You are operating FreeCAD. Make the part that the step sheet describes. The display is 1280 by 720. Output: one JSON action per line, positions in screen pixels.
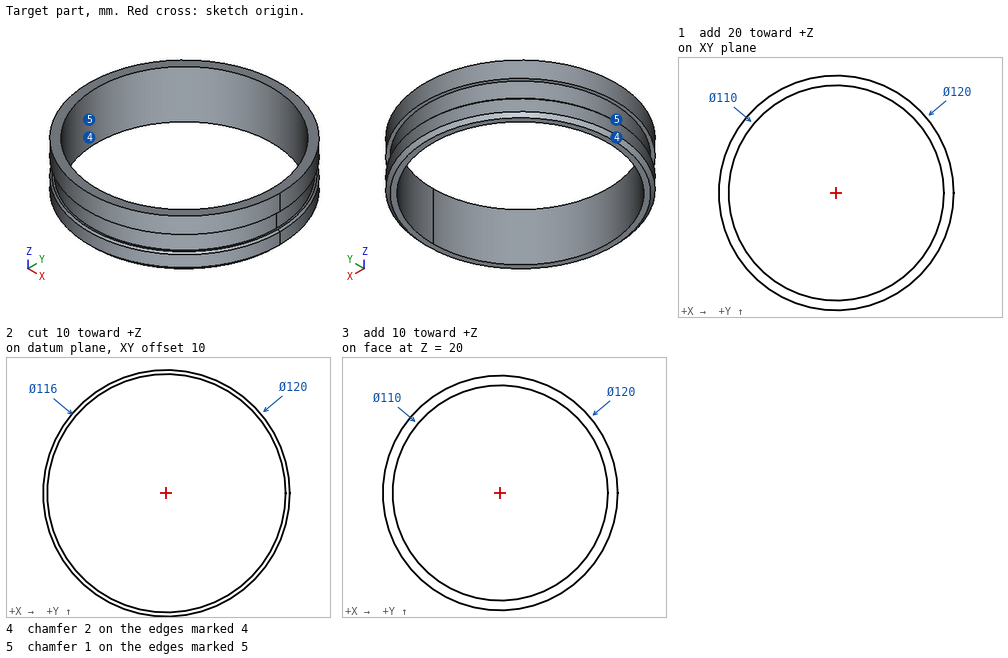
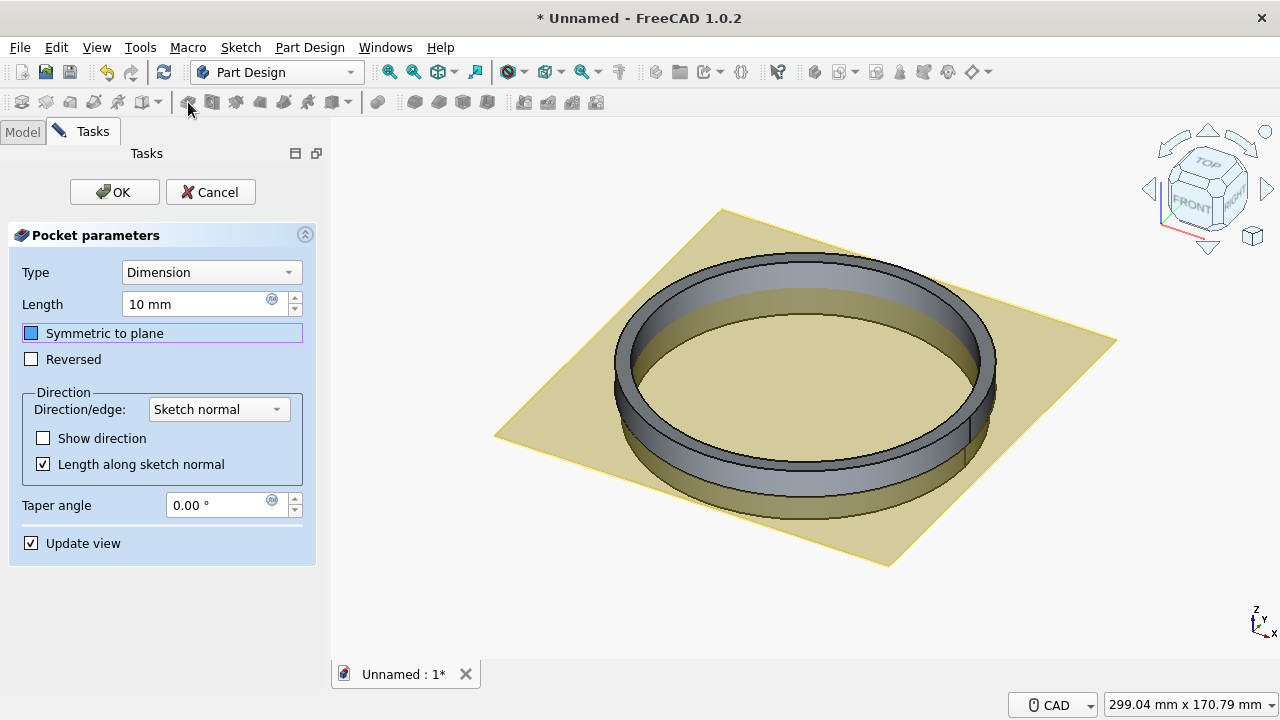
{"action": "left_click", "coordinate": [30, 359]}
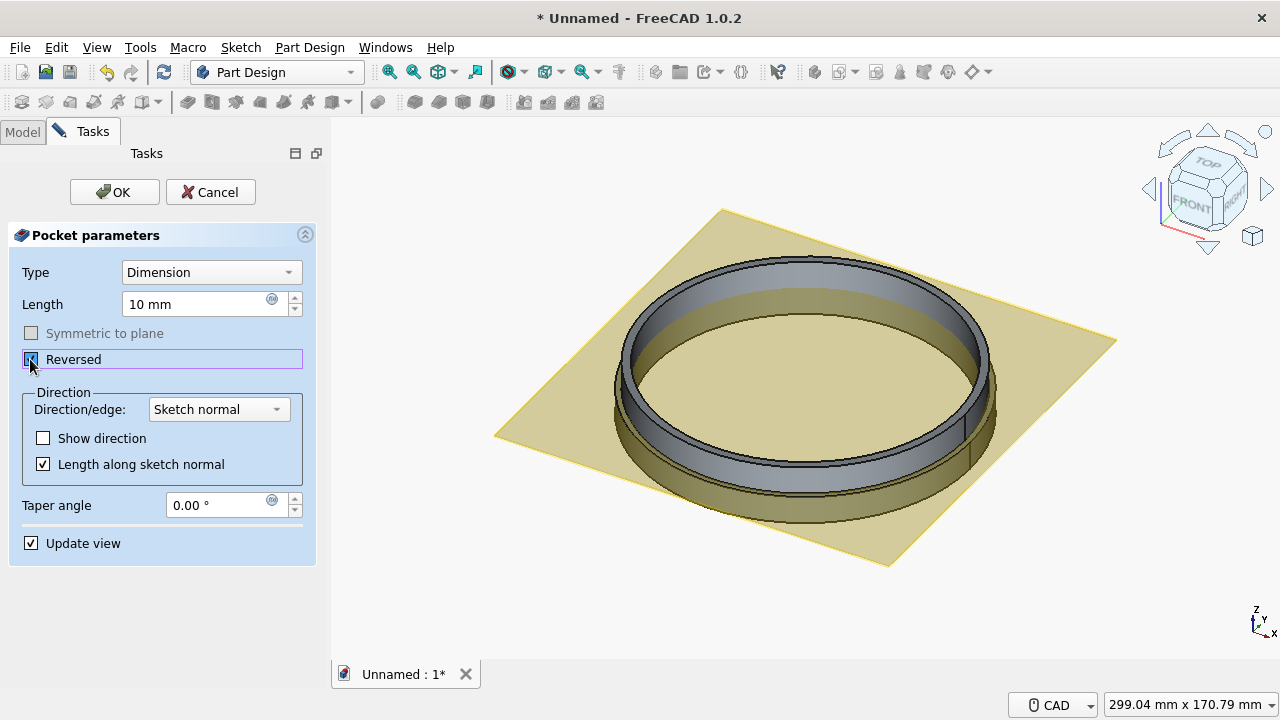
{"action": "left_click", "coordinate": [115, 192]}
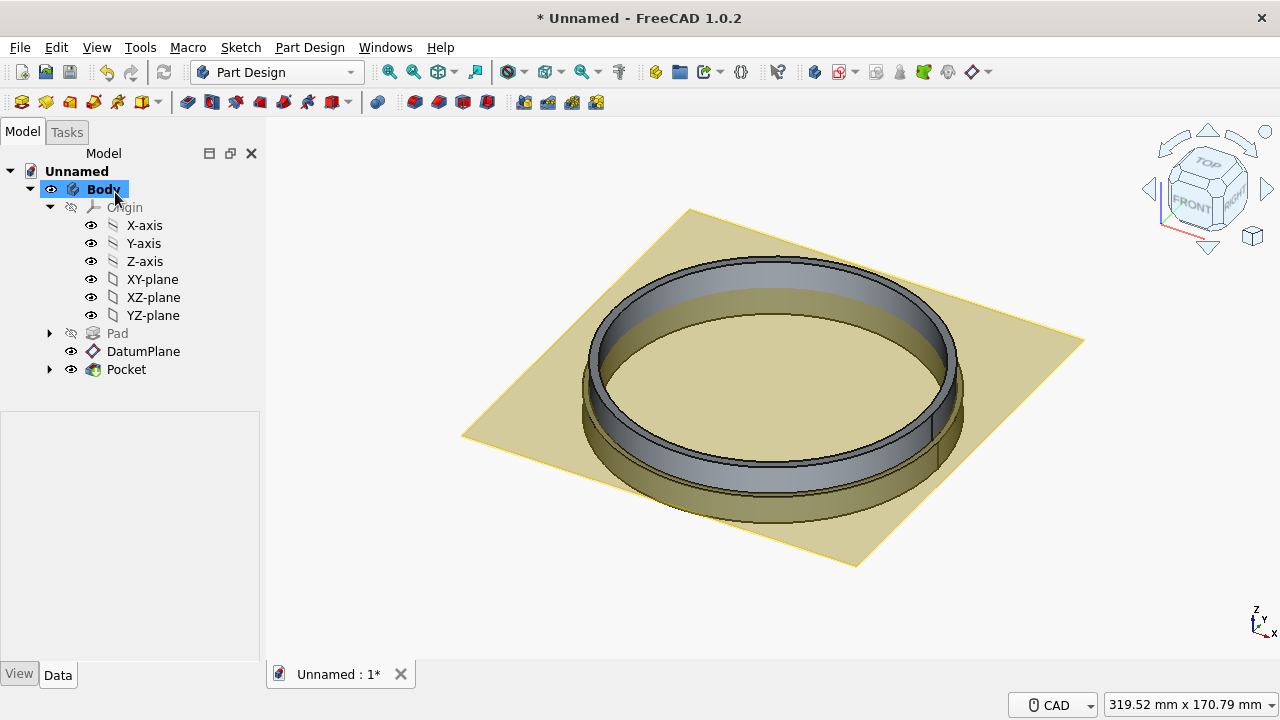
{"action": "left_click", "coordinate": [116, 351]}
{"action": "key", "text": "space"}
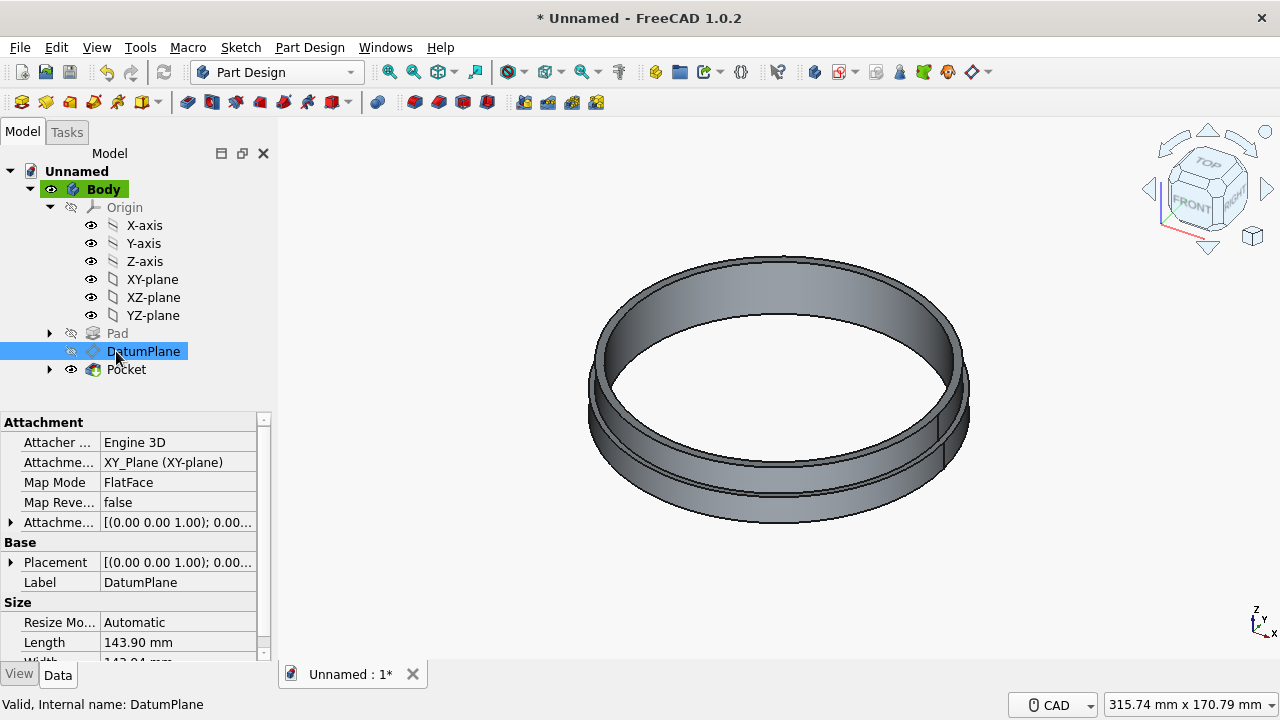
{"action": "scroll", "coordinate": [746, 463], "scroll_direction": "up", "scroll_amount": 7}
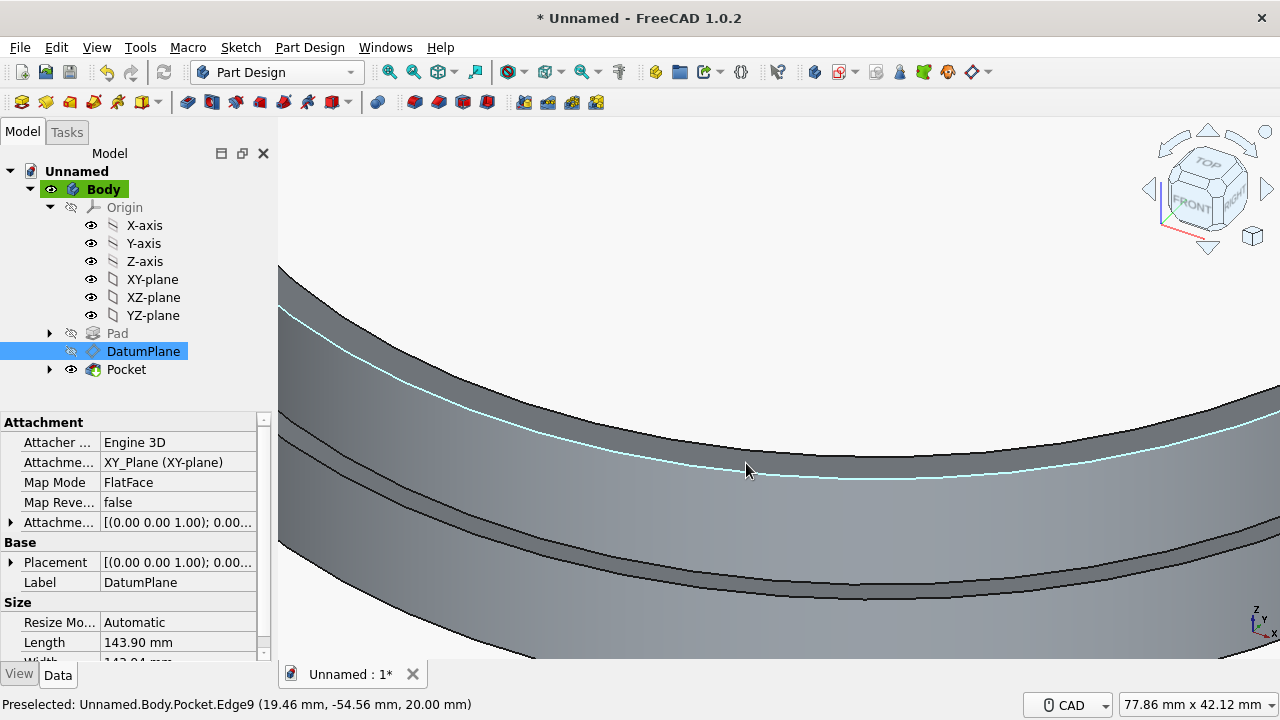
{"action": "key", "text": "v f"}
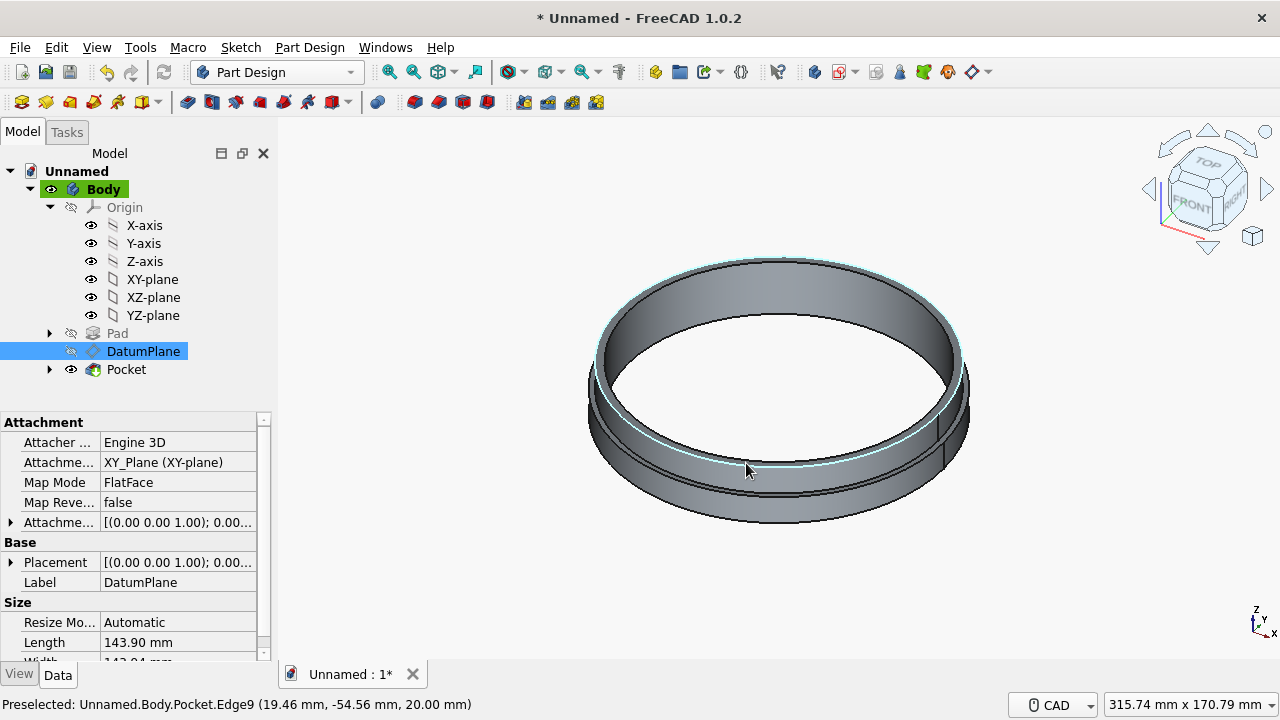
{"action": "key", "text": "0"}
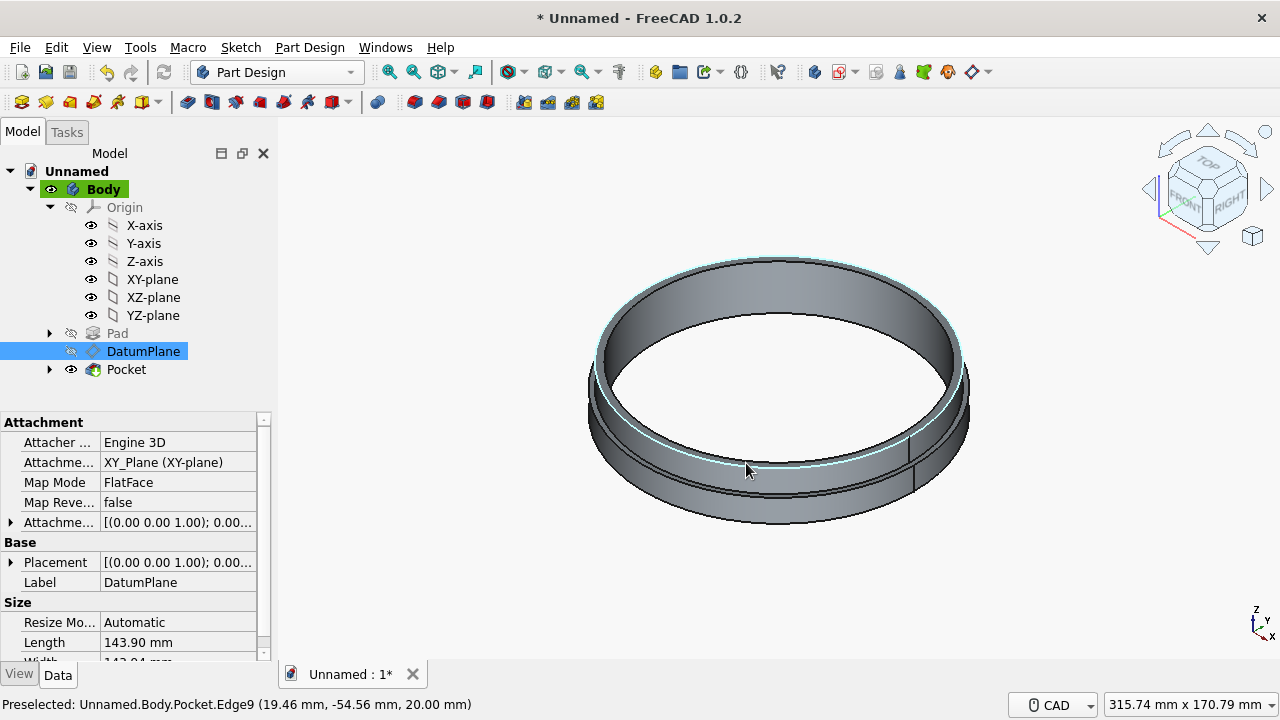
{"action": "scroll", "coordinate": [701, 455], "scroll_direction": "up", "scroll_amount": 7}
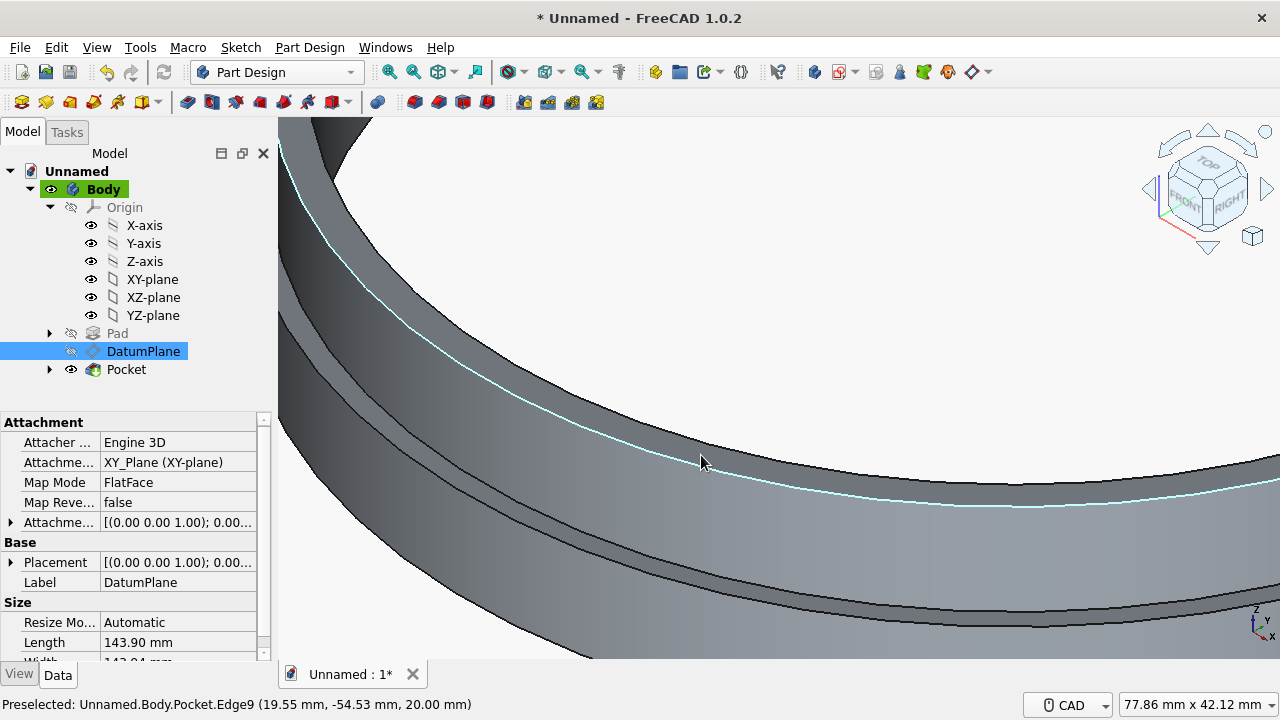
{"action": "left_click", "coordinate": [322, 212]}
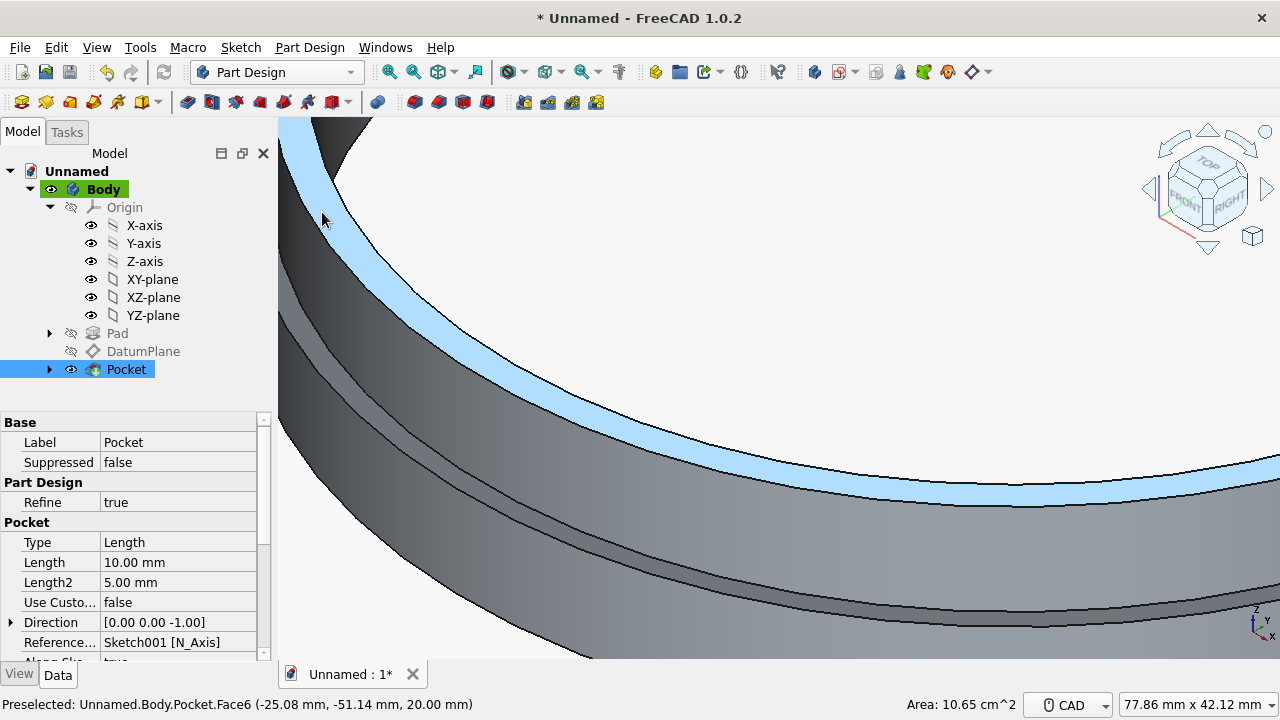
{"action": "left_click", "coordinate": [840, 72]}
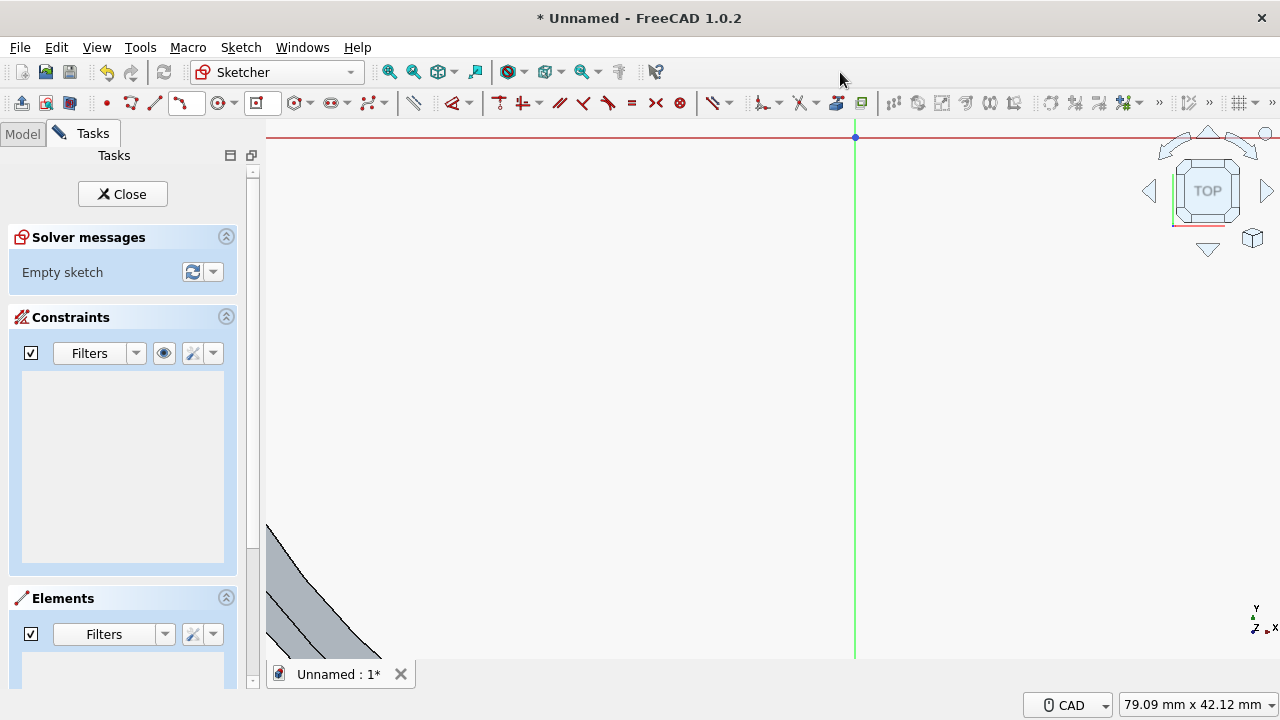
{"action": "scroll", "coordinate": [666, 452], "scroll_direction": "down", "scroll_amount": 8}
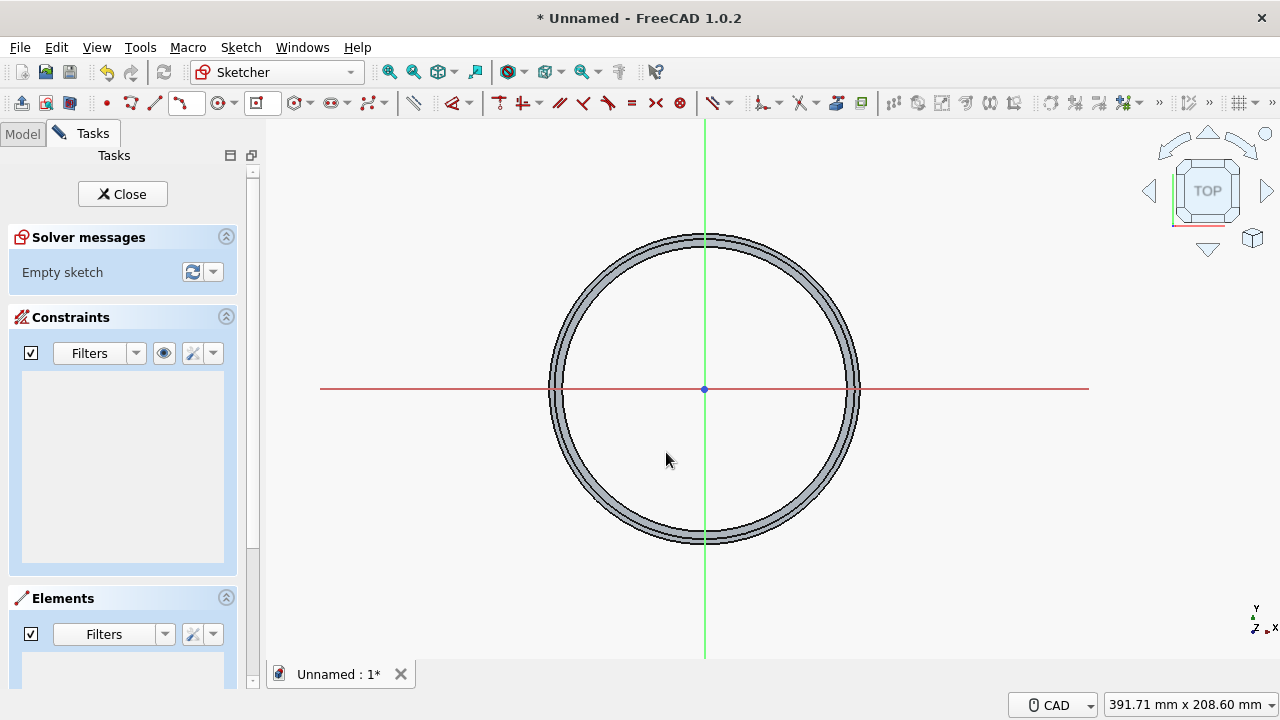
{"action": "key", "text": "g c"}